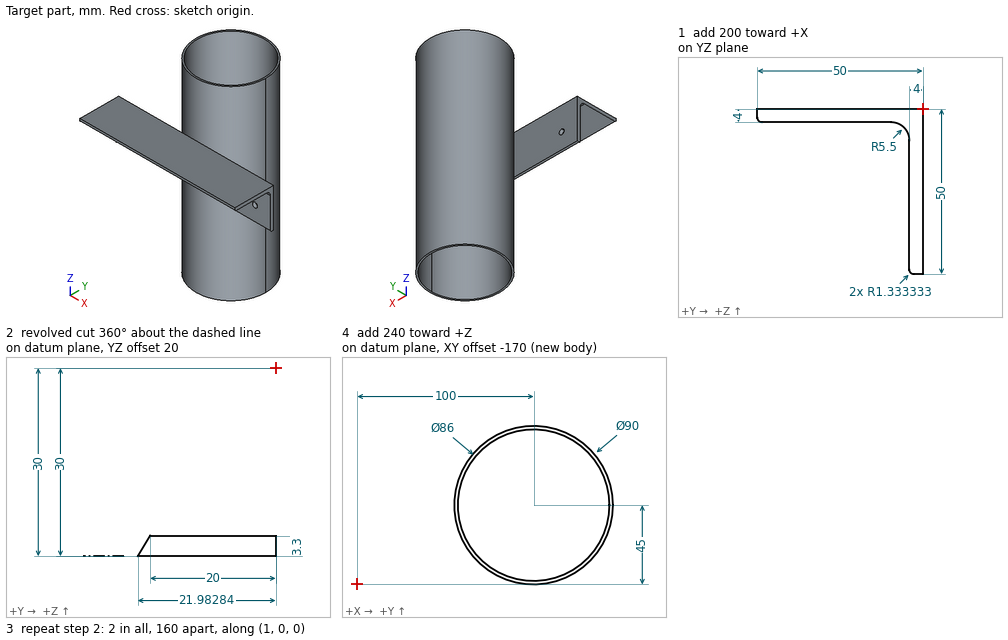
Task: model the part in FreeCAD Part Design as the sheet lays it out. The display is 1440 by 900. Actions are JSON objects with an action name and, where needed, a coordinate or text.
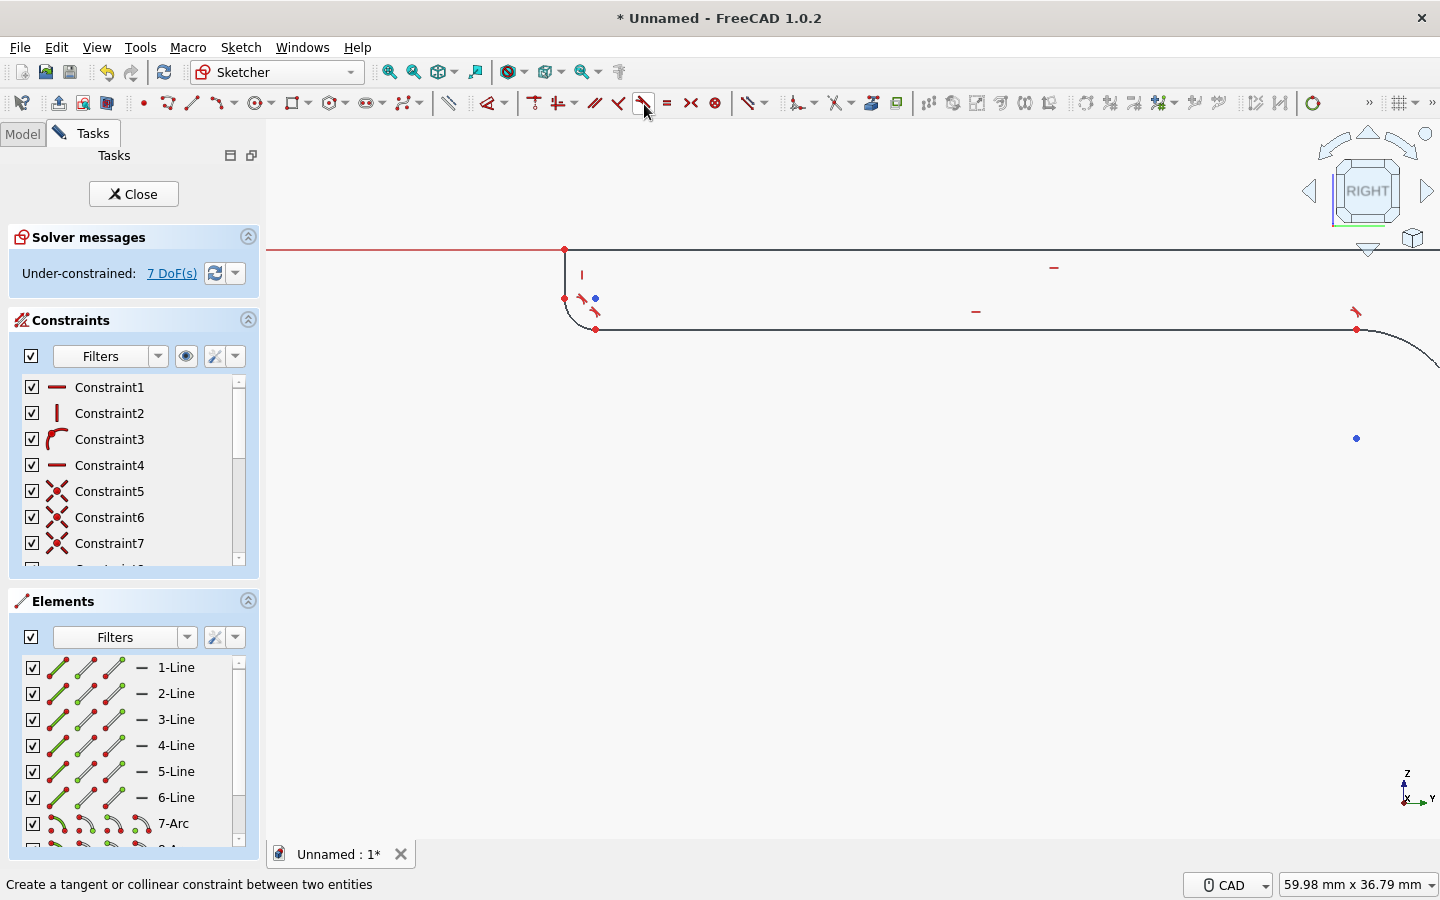
{"action": "scroll", "coordinate": [564, 267], "scroll_direction": "down", "scroll_amount": 4}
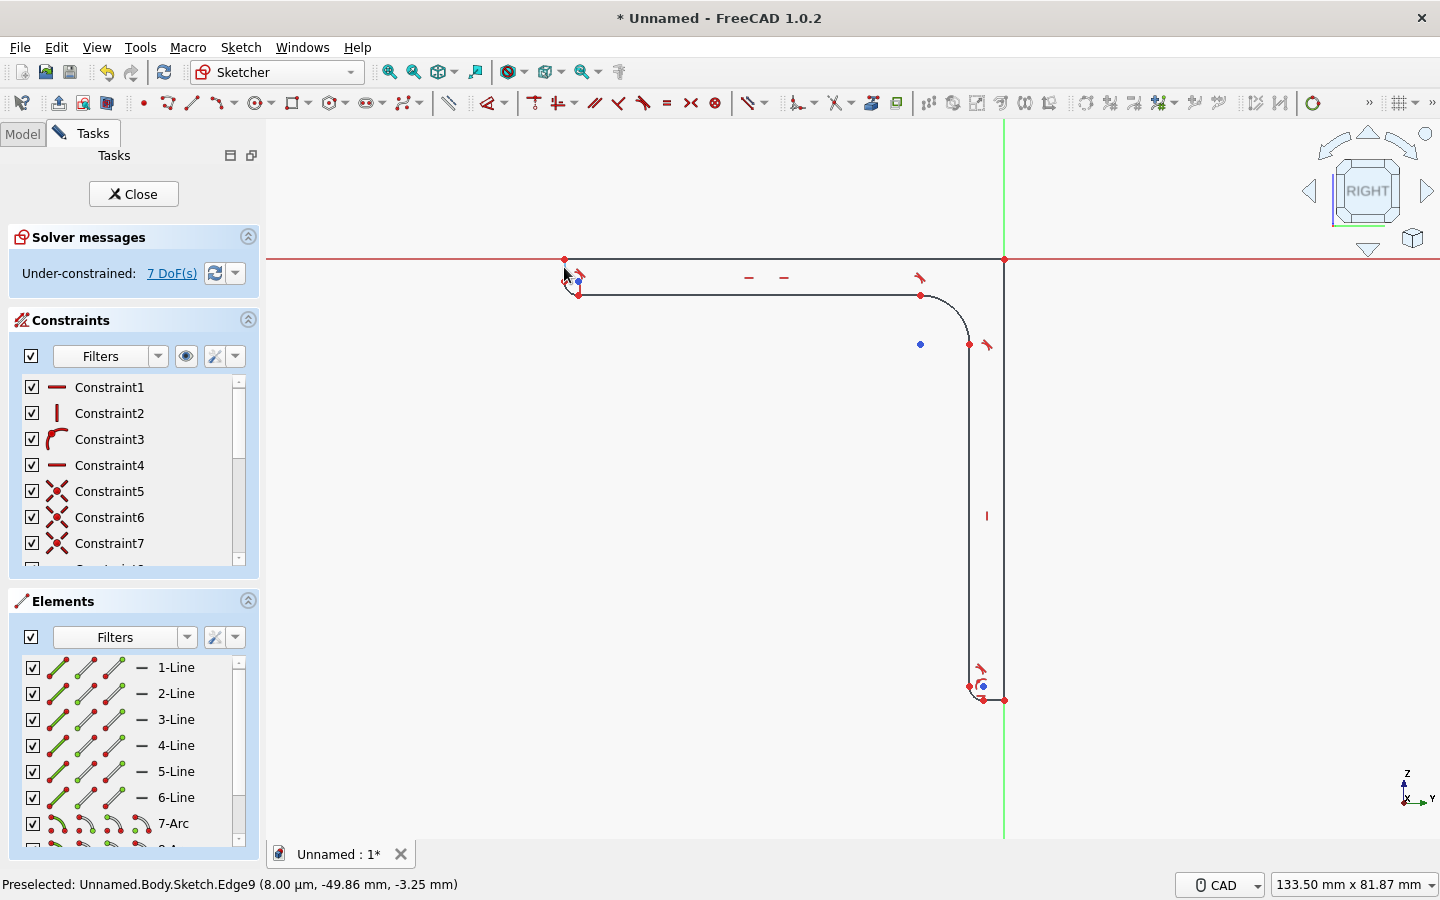
{"action": "scroll", "coordinate": [971, 693], "scroll_direction": "up", "scroll_amount": 4}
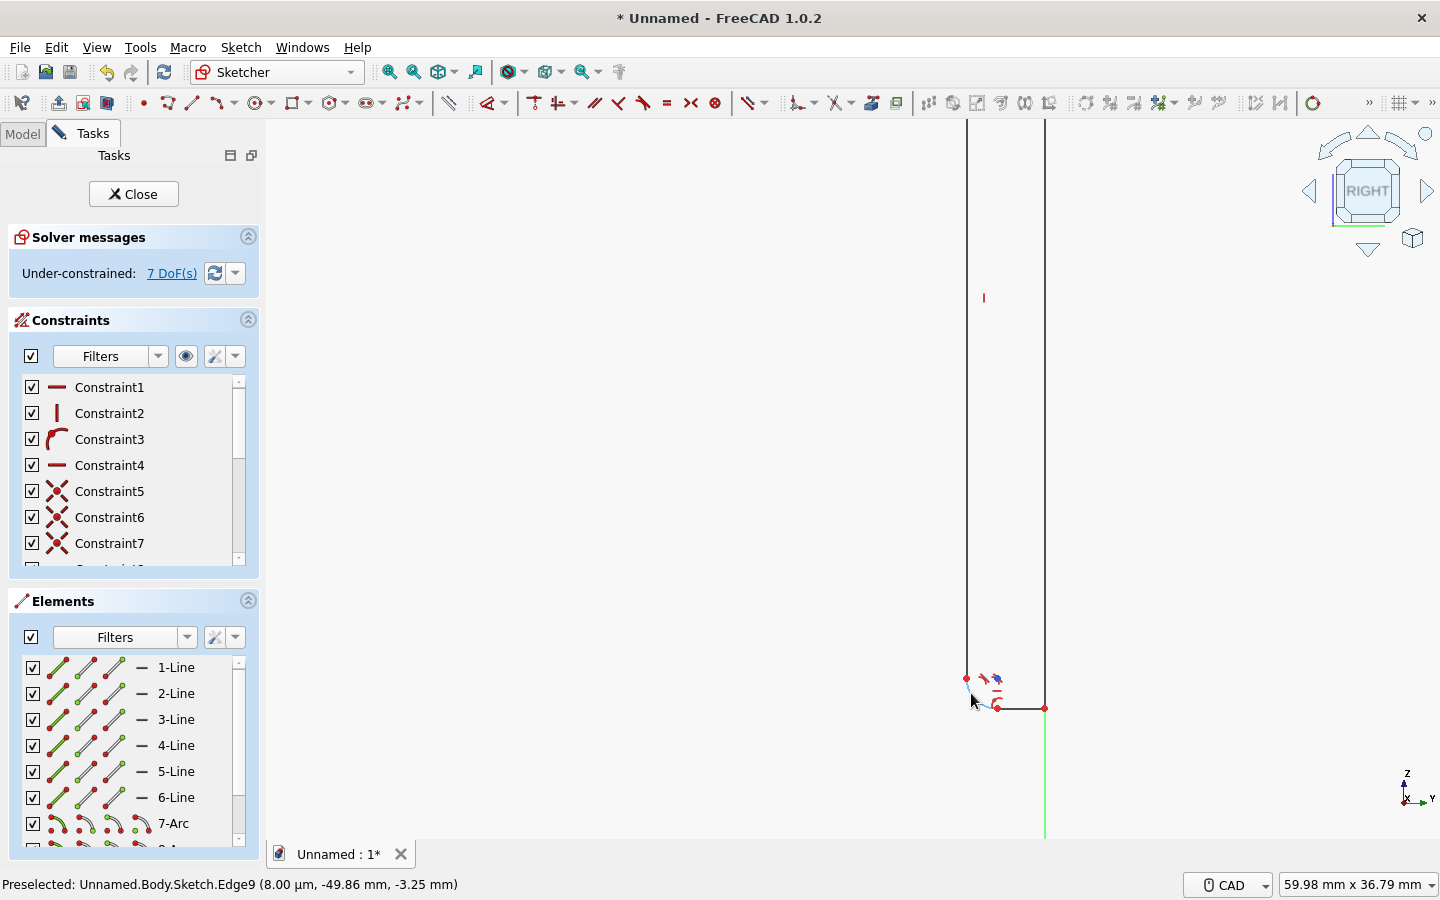
{"action": "left_click", "coordinate": [970, 692]}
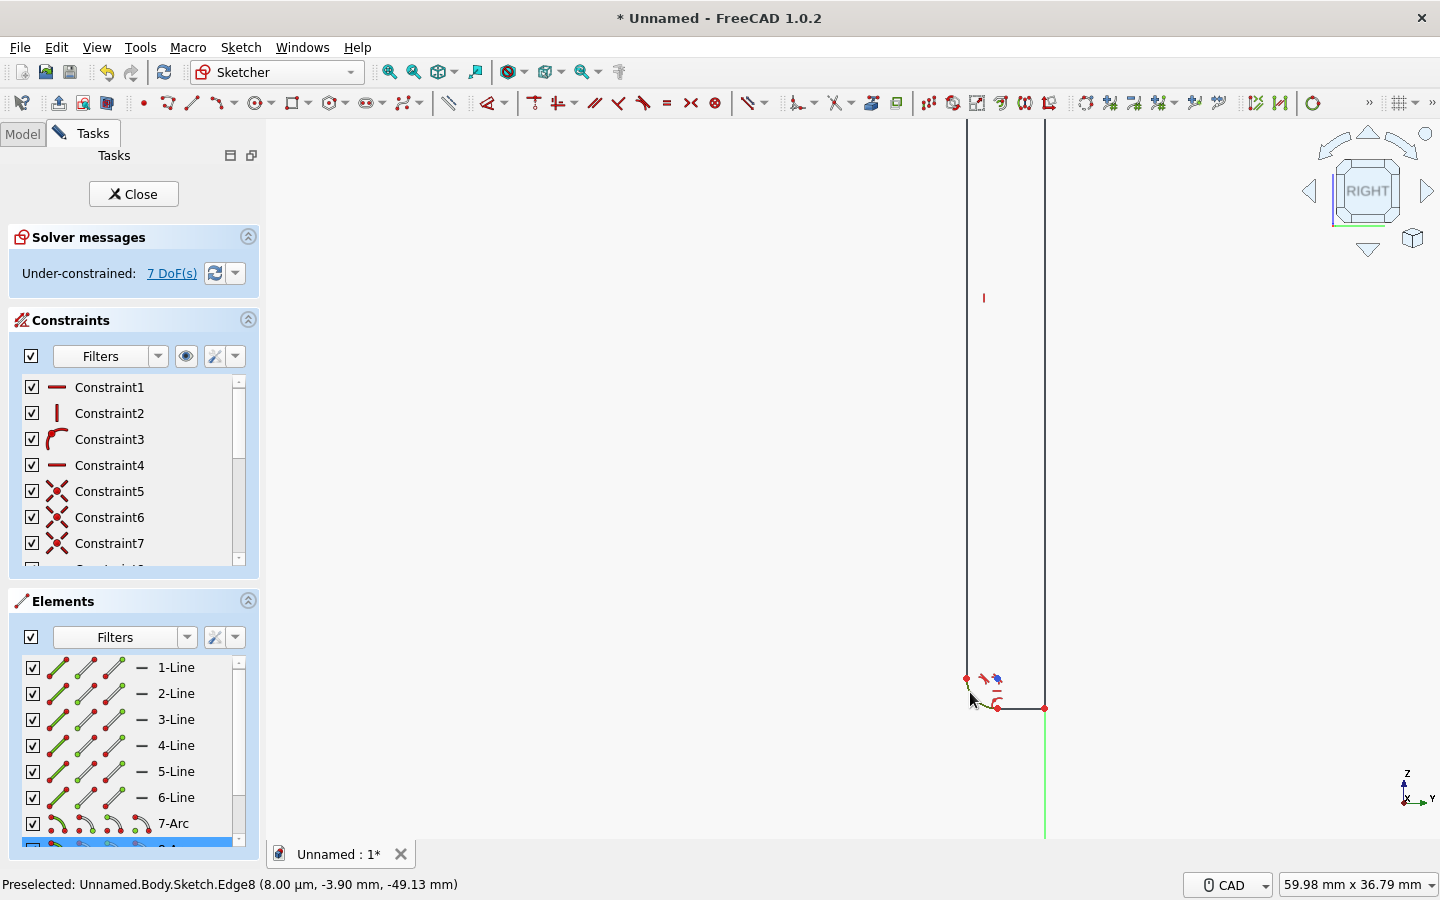
{"action": "scroll", "coordinate": [971, 693], "scroll_direction": "down", "scroll_amount": 4}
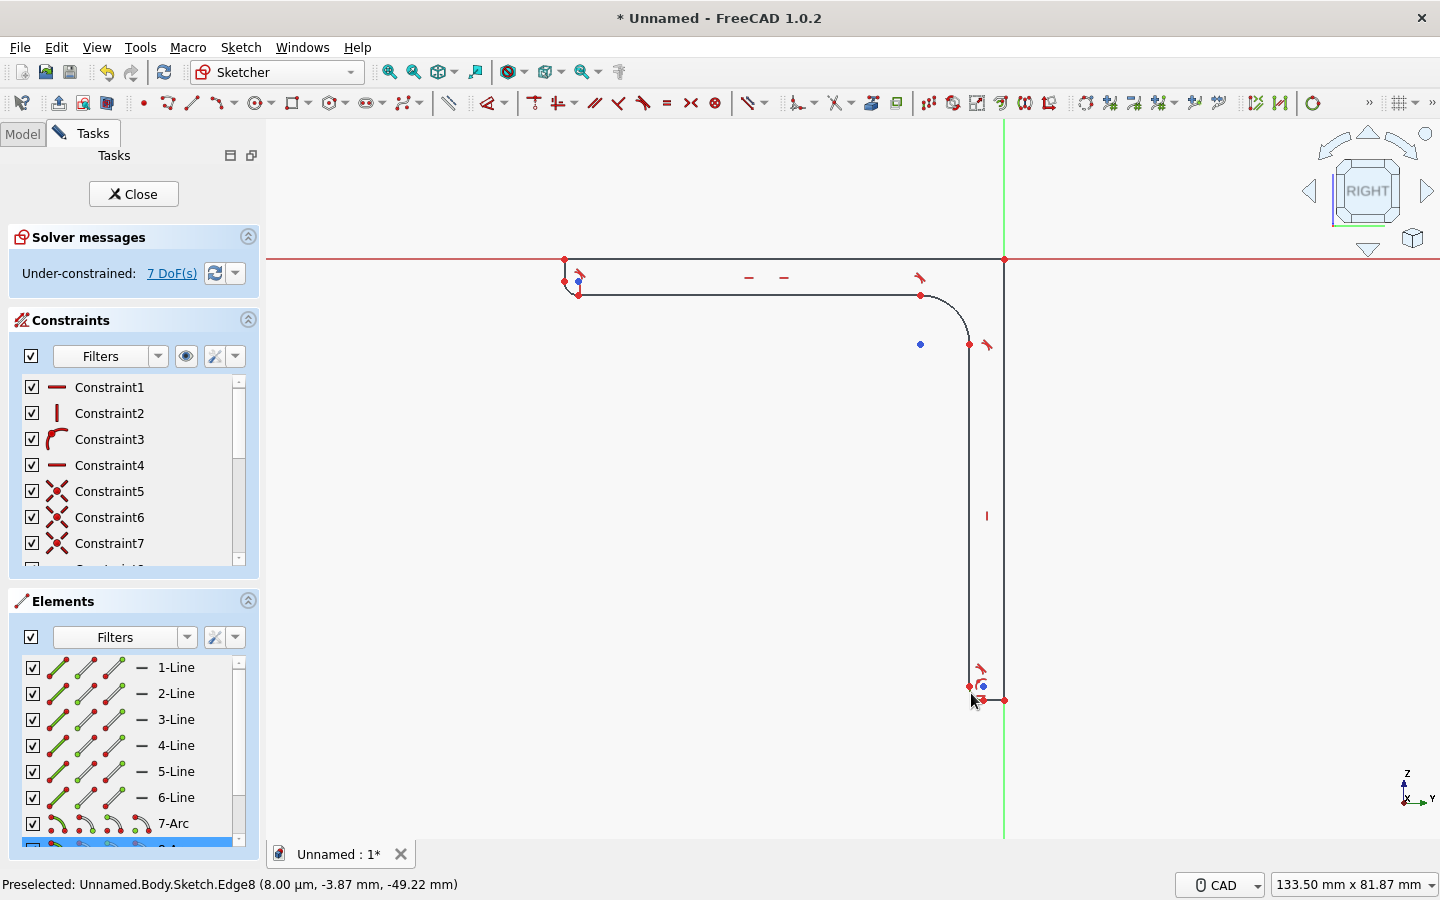
{"action": "scroll", "coordinate": [566, 288], "scroll_direction": "up", "scroll_amount": 4}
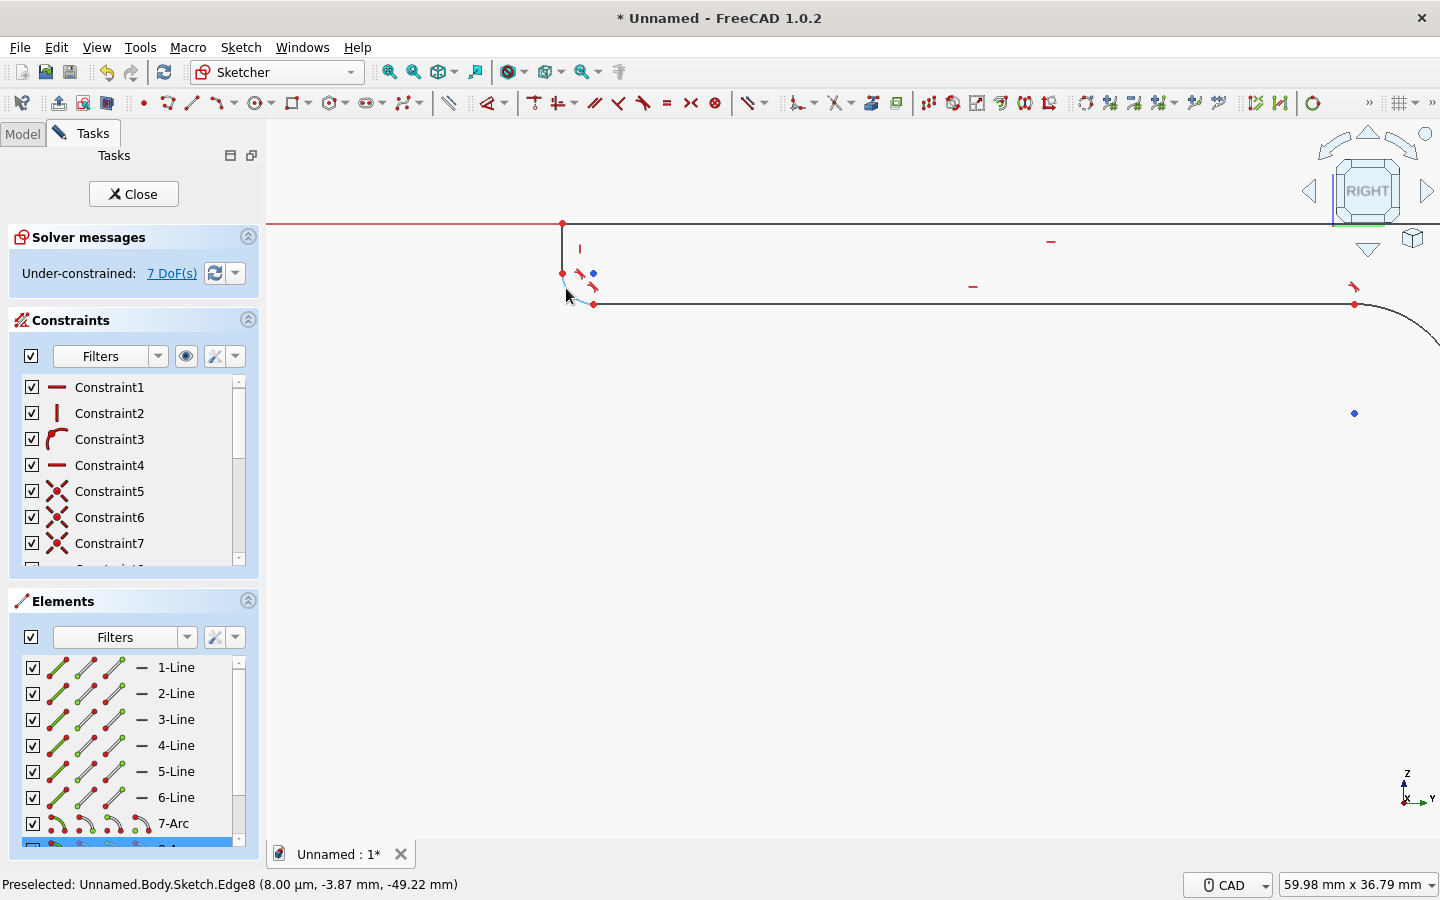
{"action": "left_click", "coordinate": [566, 287]}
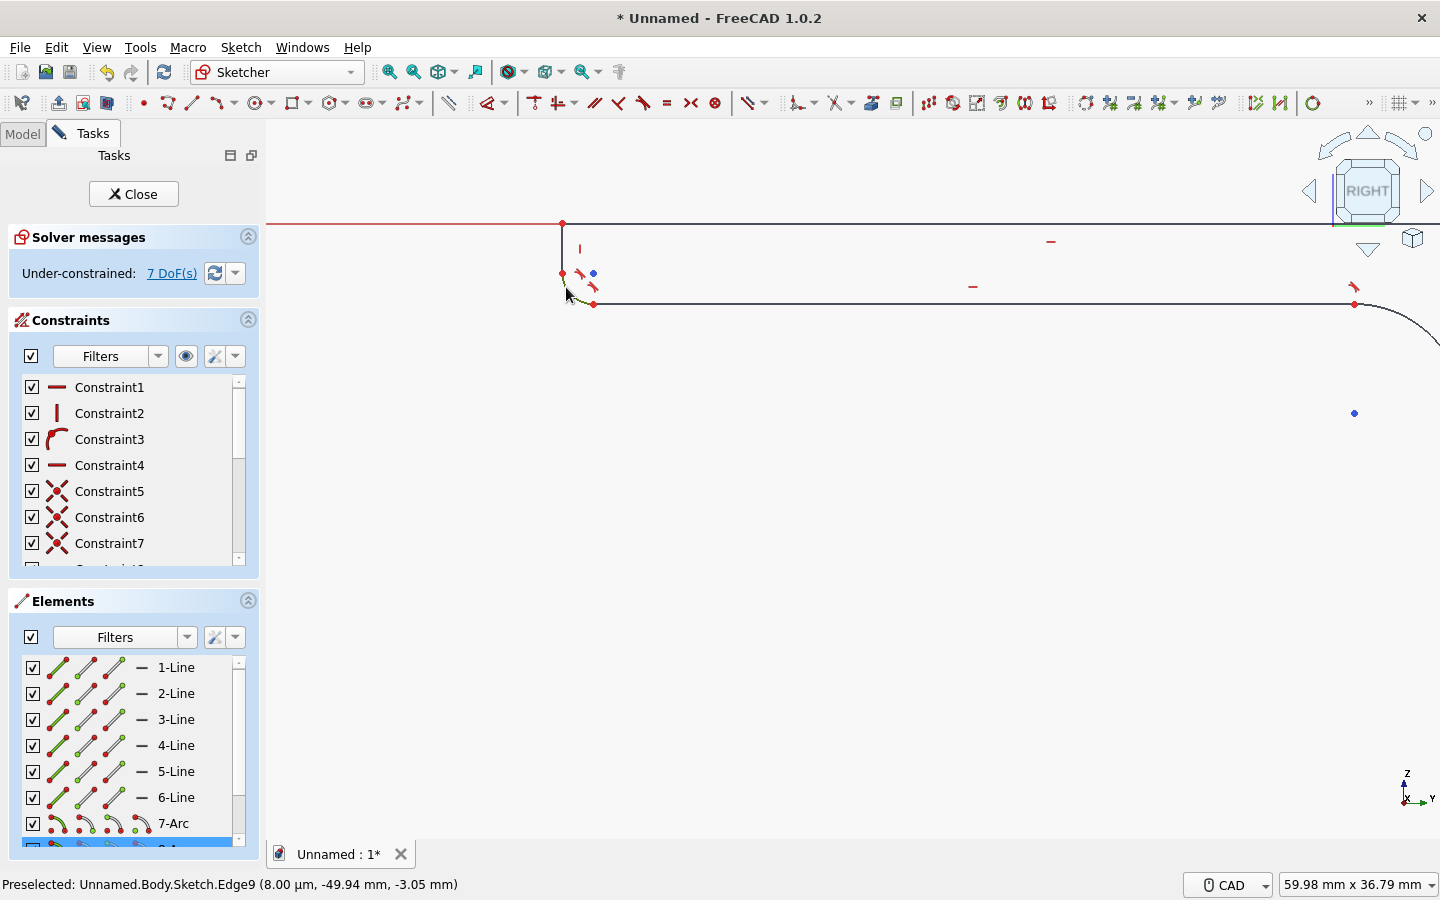
{"action": "left_click", "coordinate": [668, 104]}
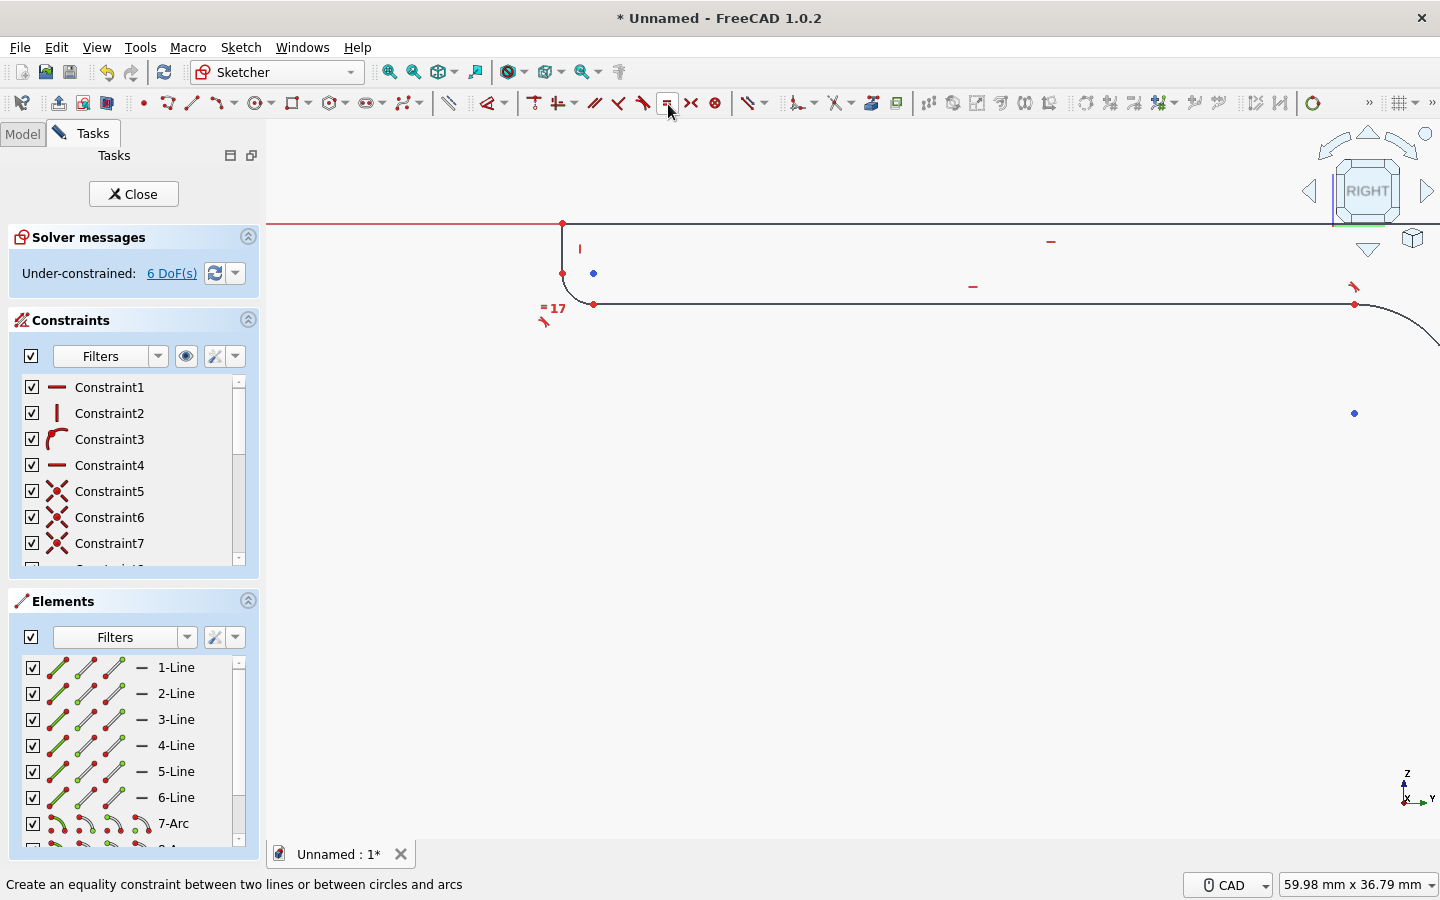
{"action": "scroll", "coordinate": [566, 288], "scroll_direction": "down", "scroll_amount": 4}